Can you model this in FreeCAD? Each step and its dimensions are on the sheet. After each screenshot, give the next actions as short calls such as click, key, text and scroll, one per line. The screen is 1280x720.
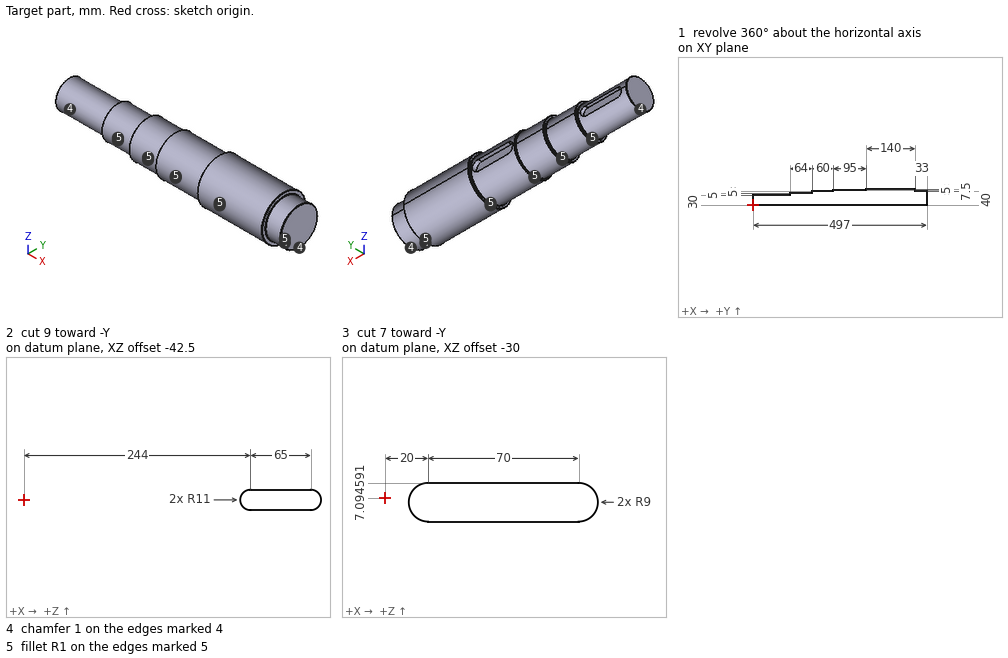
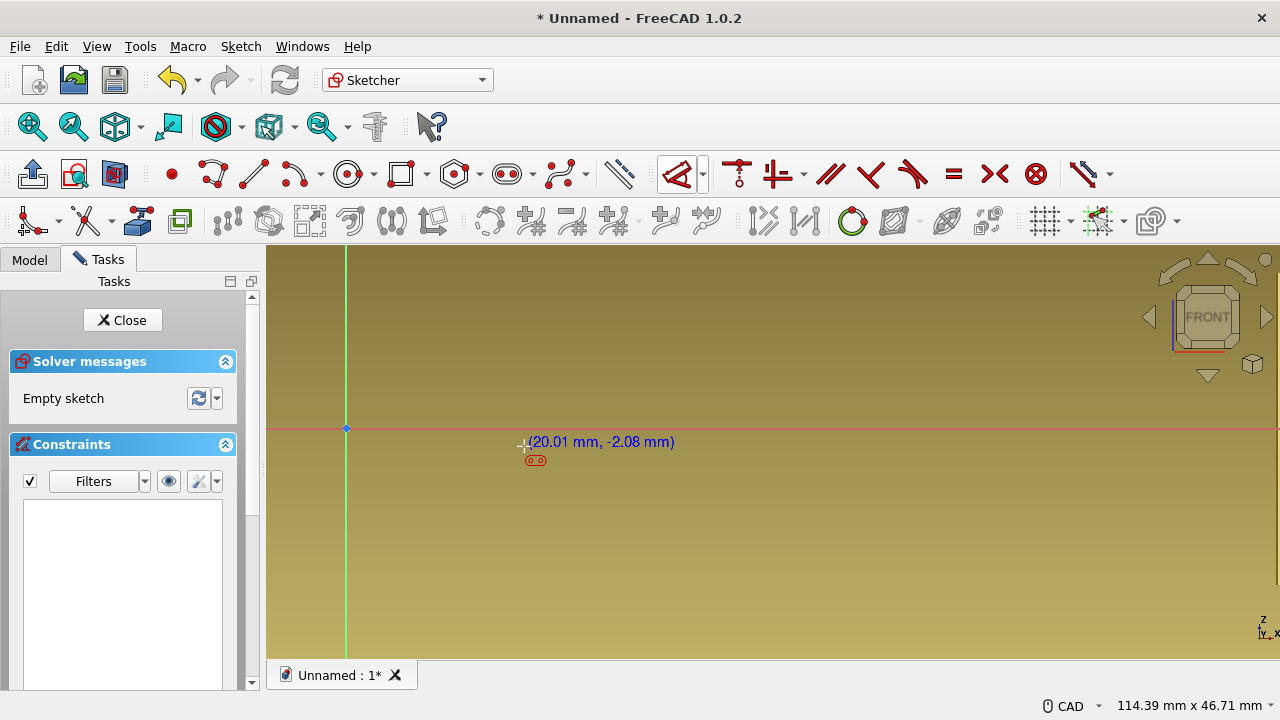
click(524, 446)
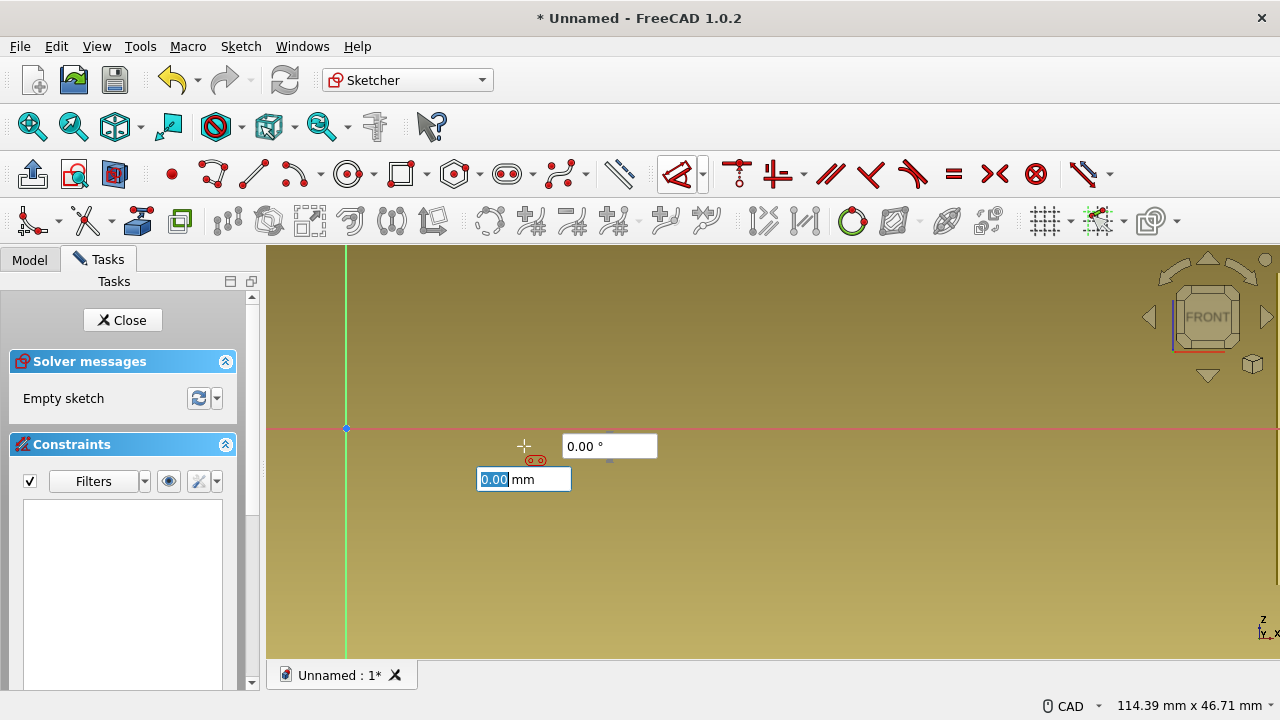
scroll(540, 465, down, 2)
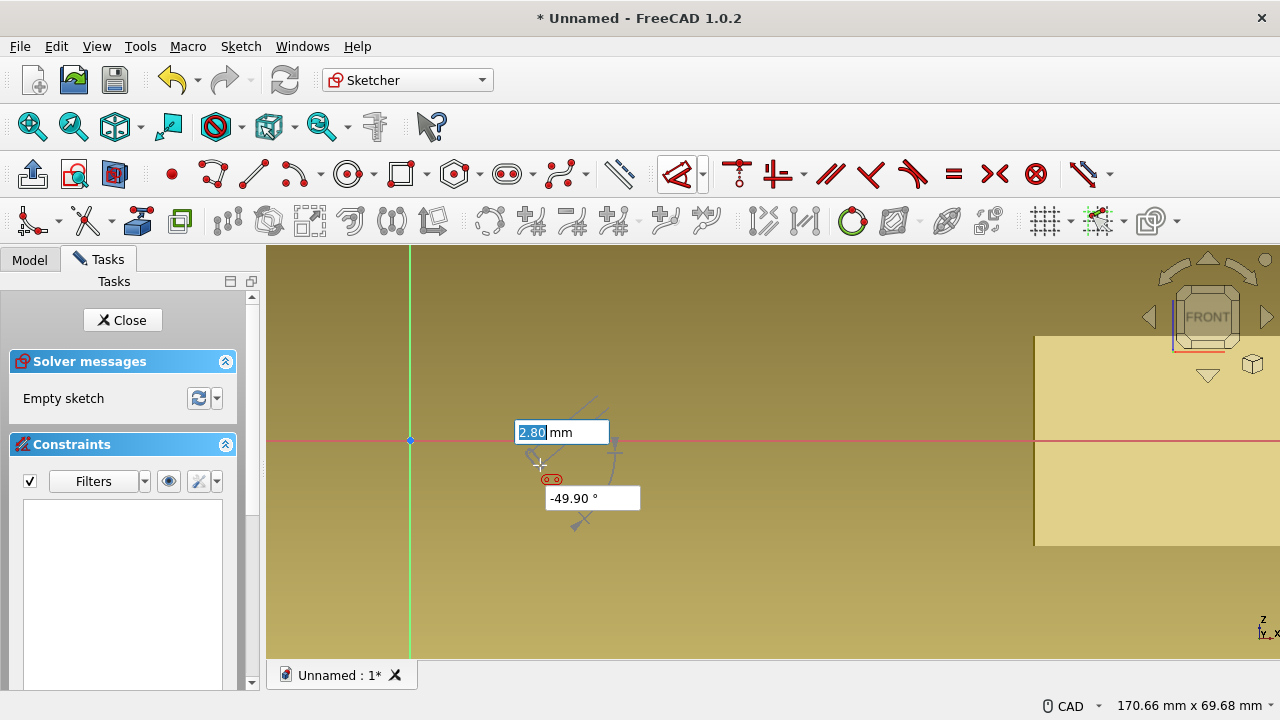
scroll(945, 452, up, 2)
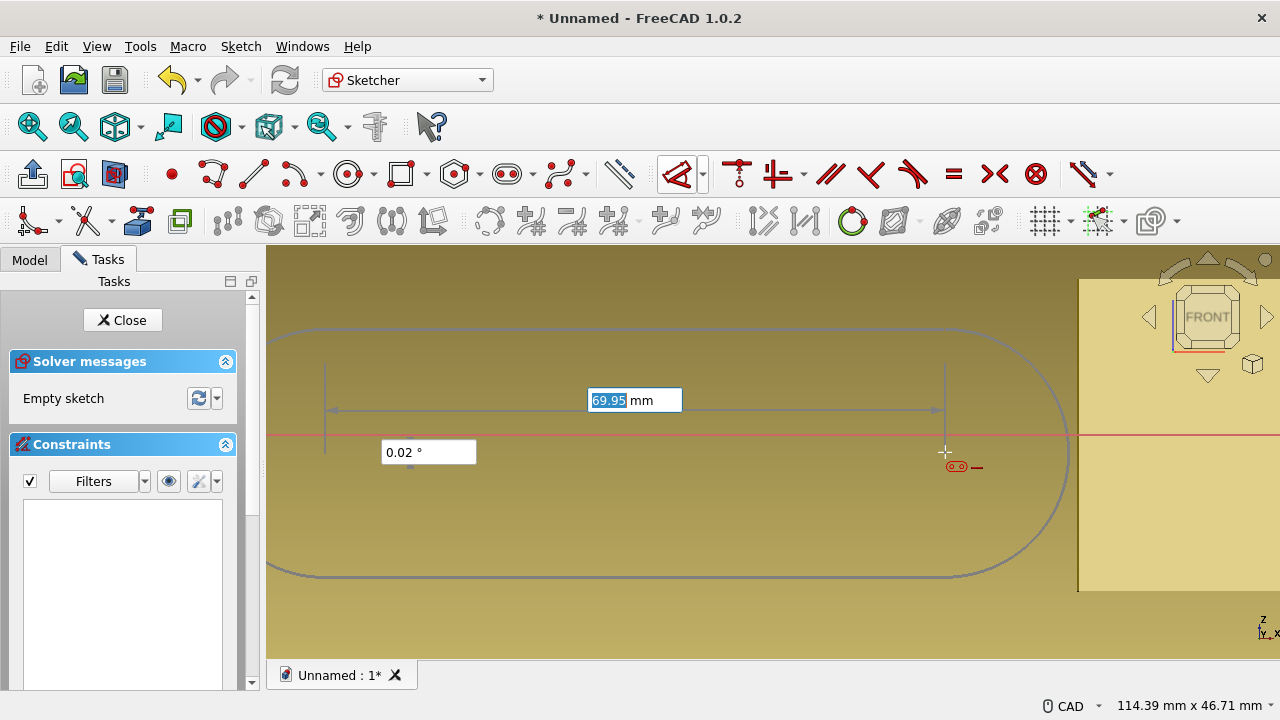
click(945, 452)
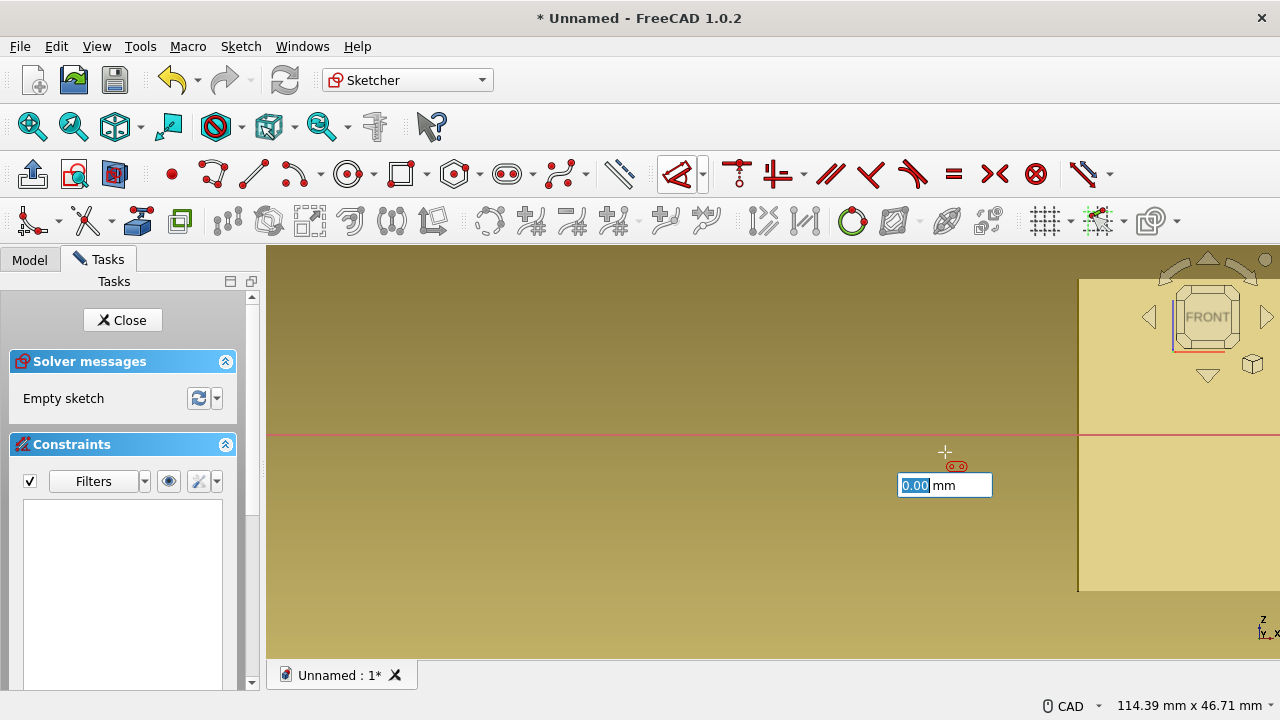
click(635, 532)
key(Escape)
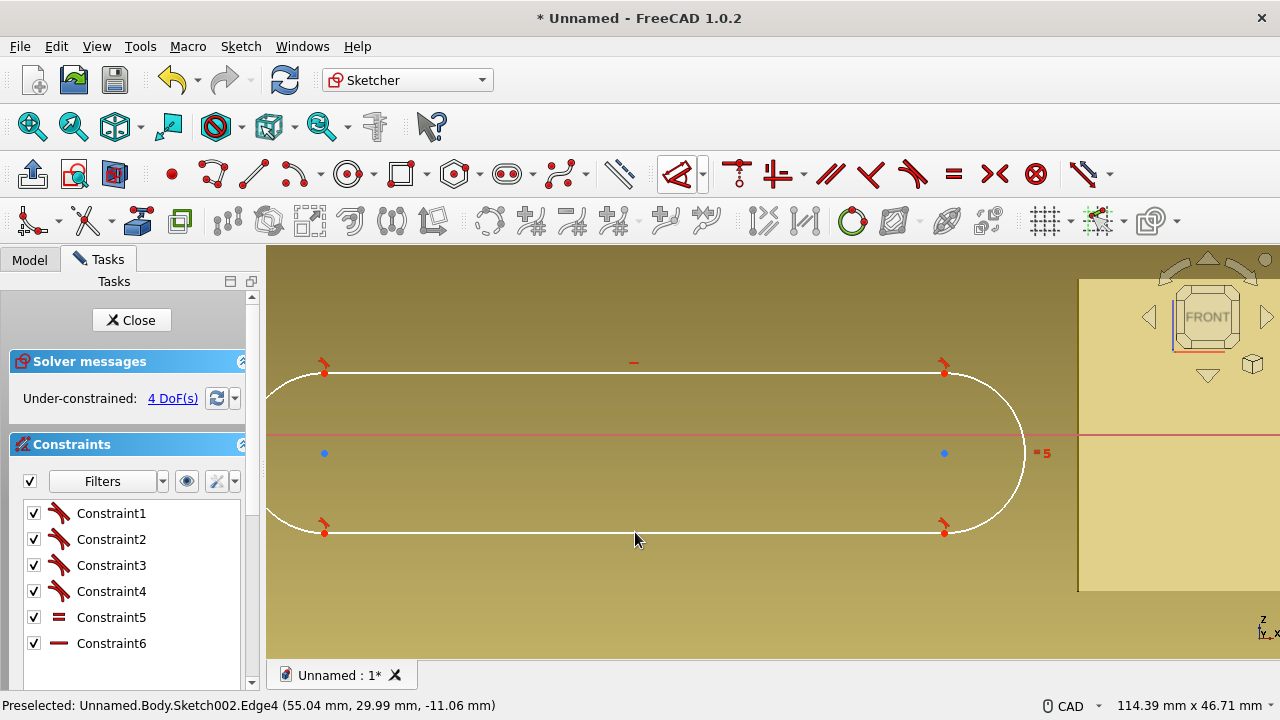
scroll(946, 452, down, 2)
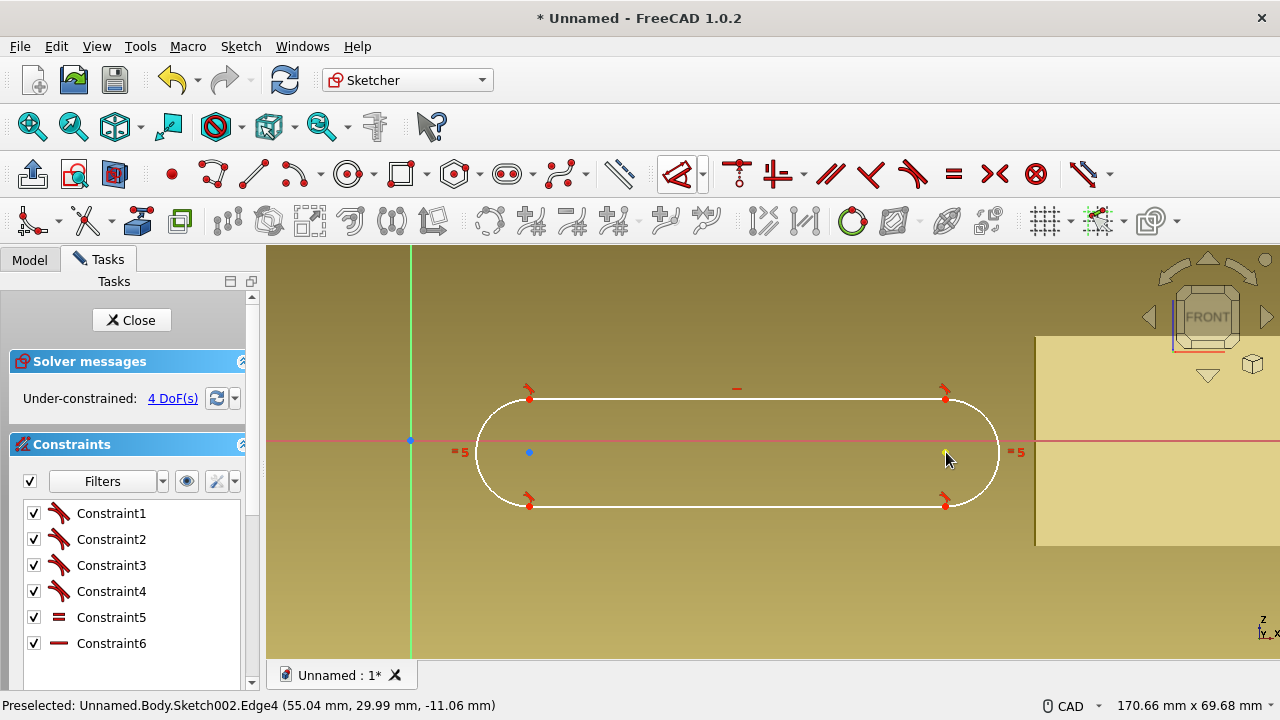
click(486, 421)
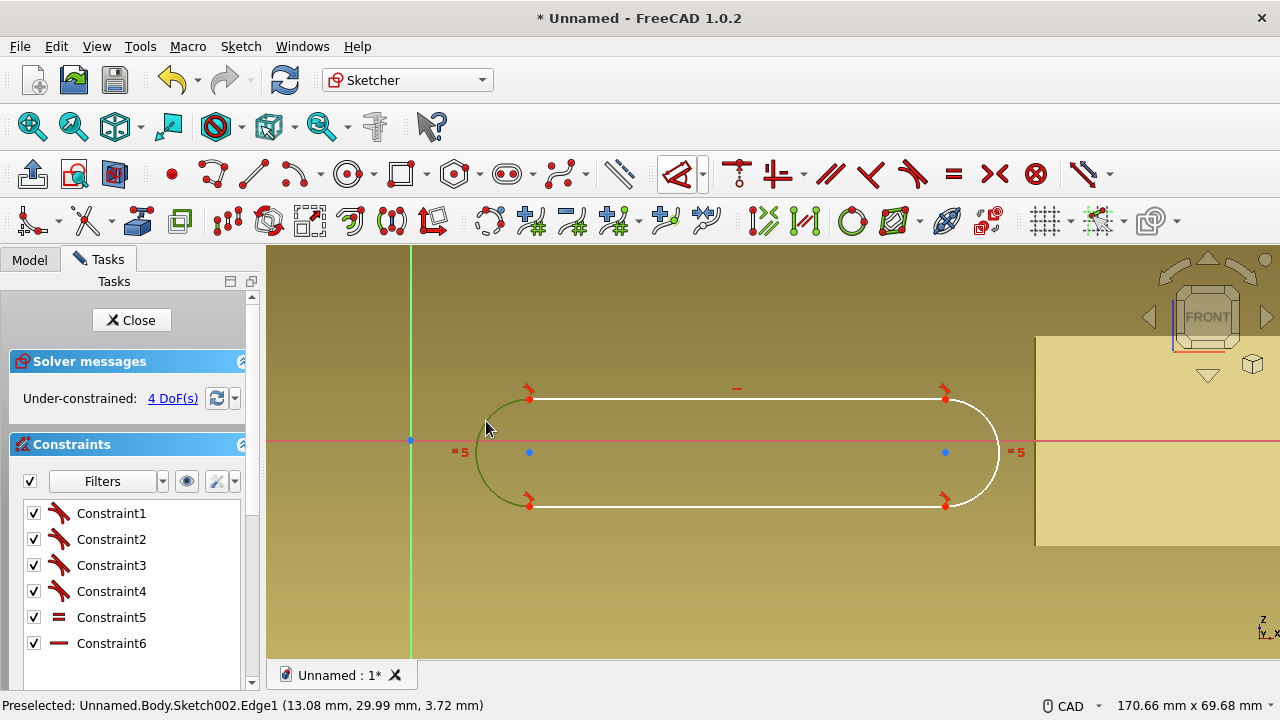
click(702, 174)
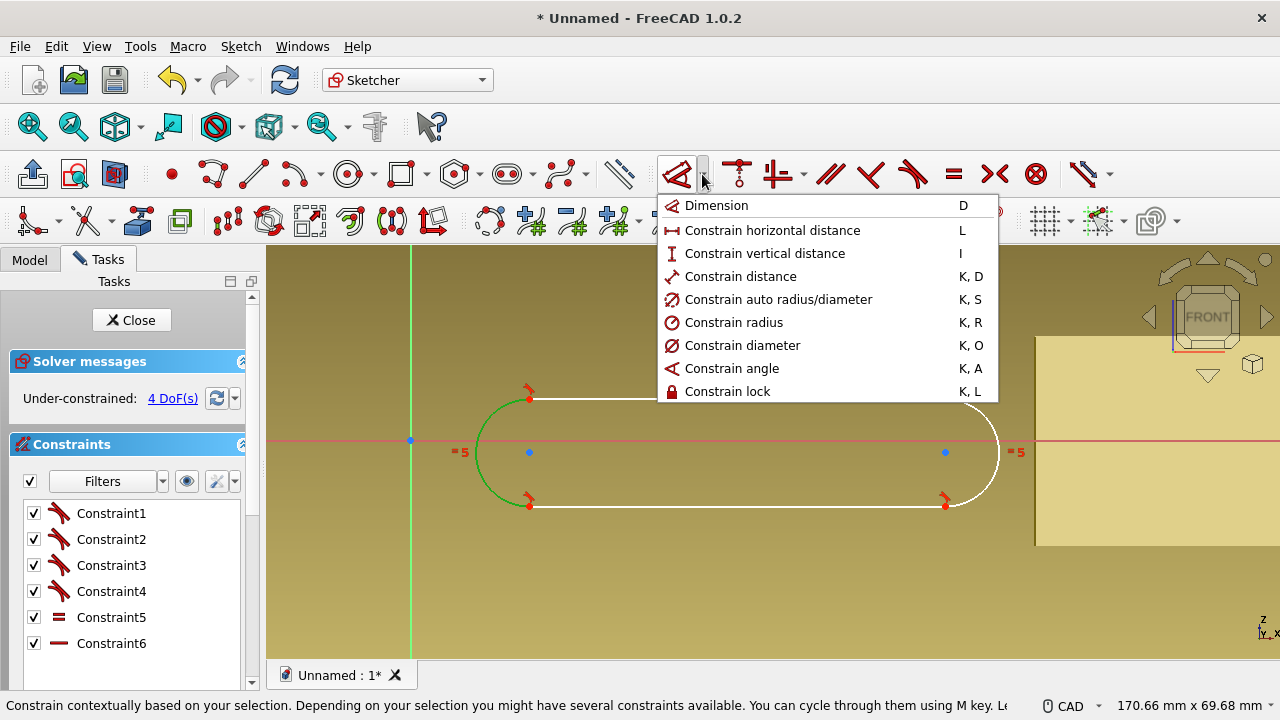
click(828, 322)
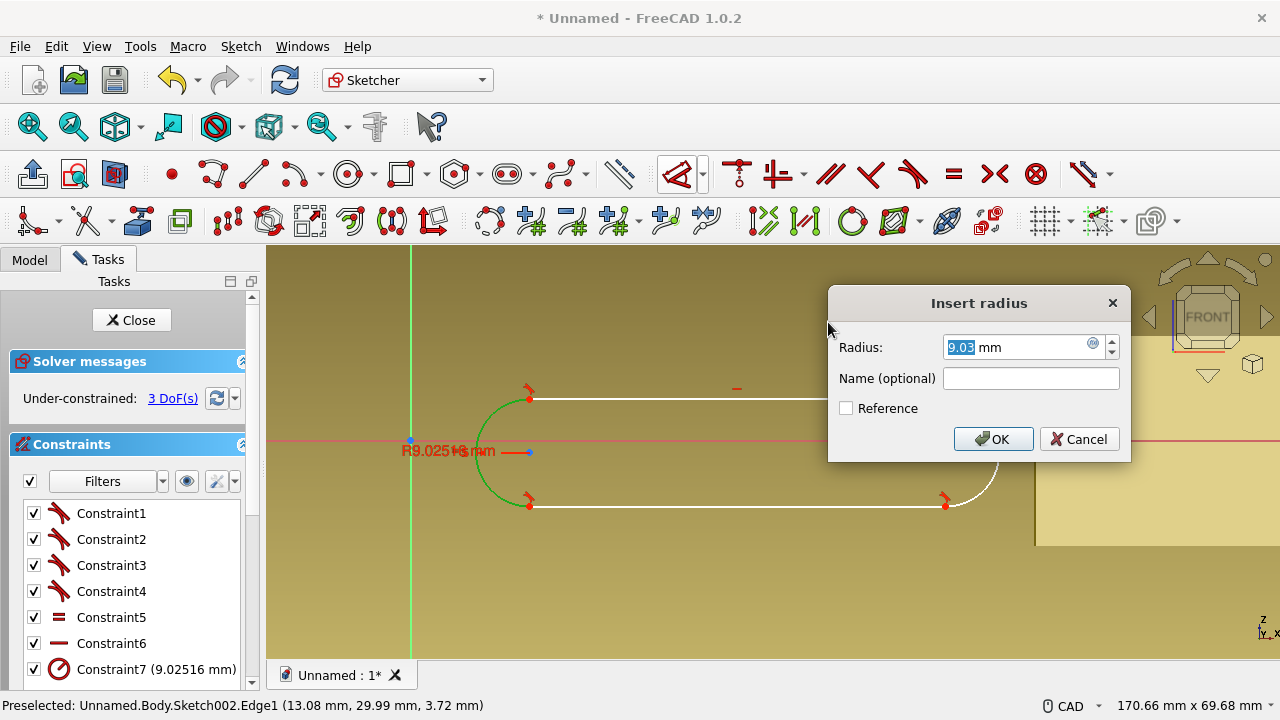
text(9)
key(Return)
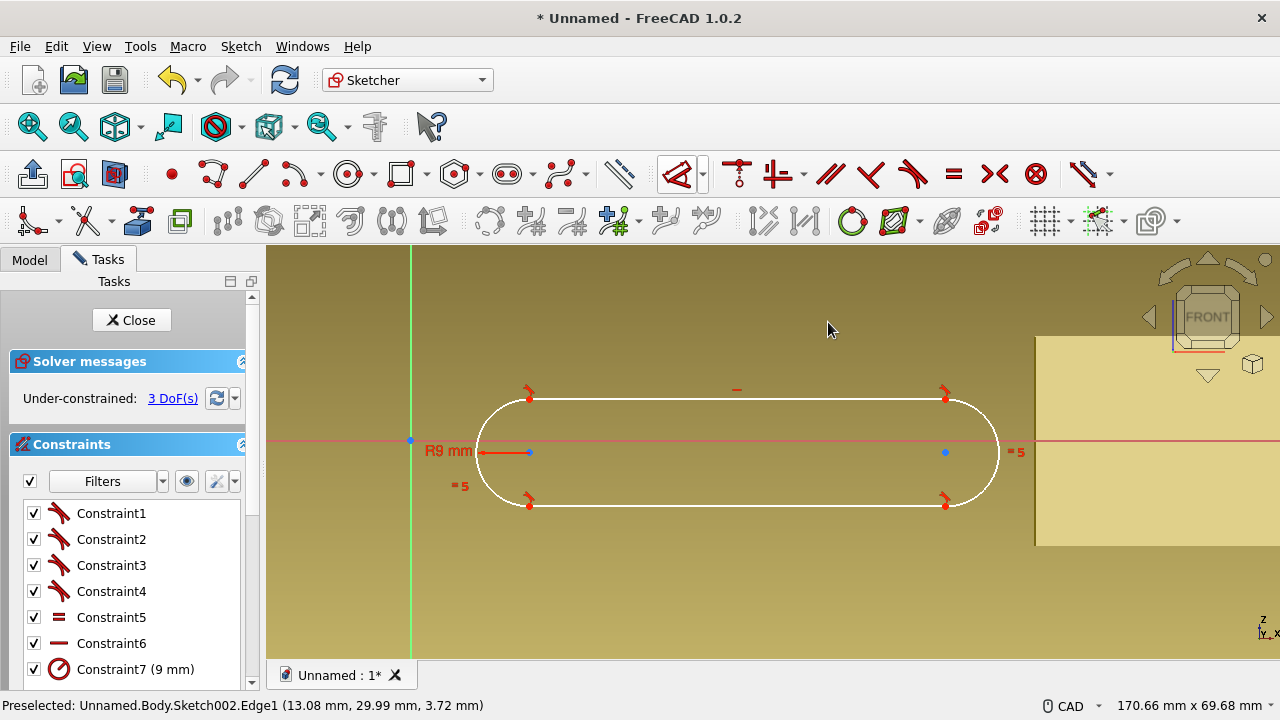
click(654, 399)